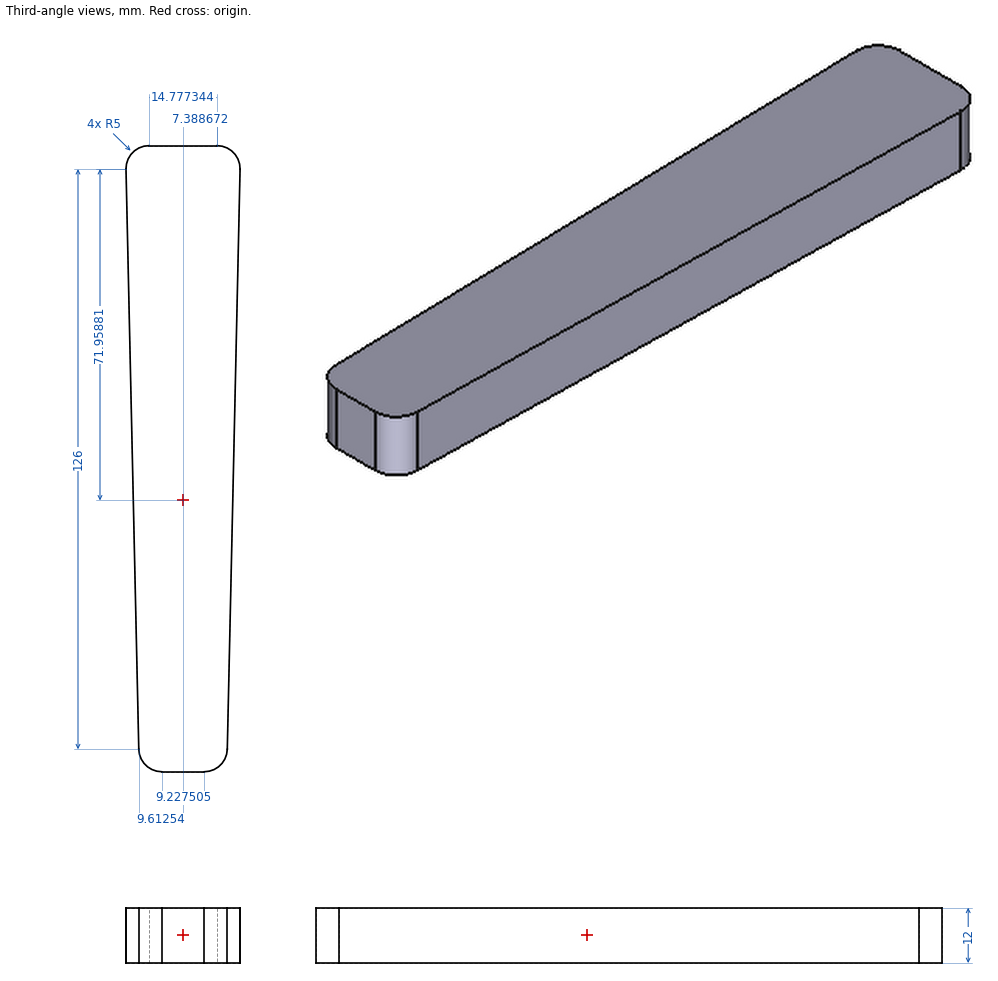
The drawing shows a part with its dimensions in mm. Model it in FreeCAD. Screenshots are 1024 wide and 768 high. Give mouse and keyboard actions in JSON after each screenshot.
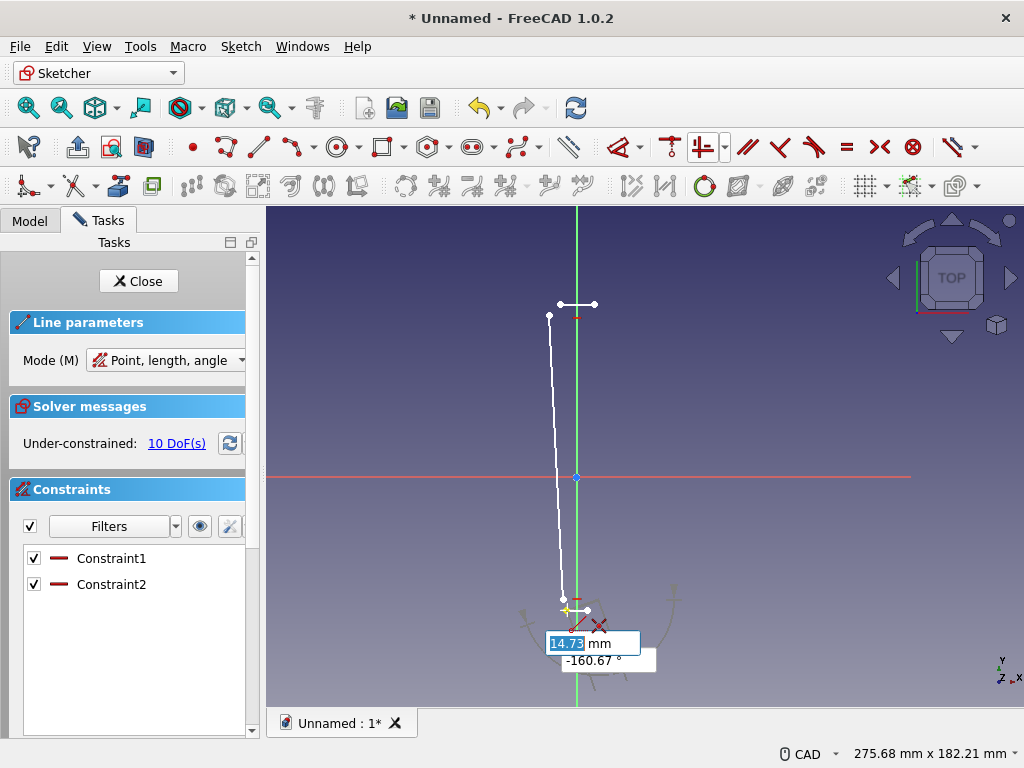
{"action": "left_click", "coordinate": [613, 315]}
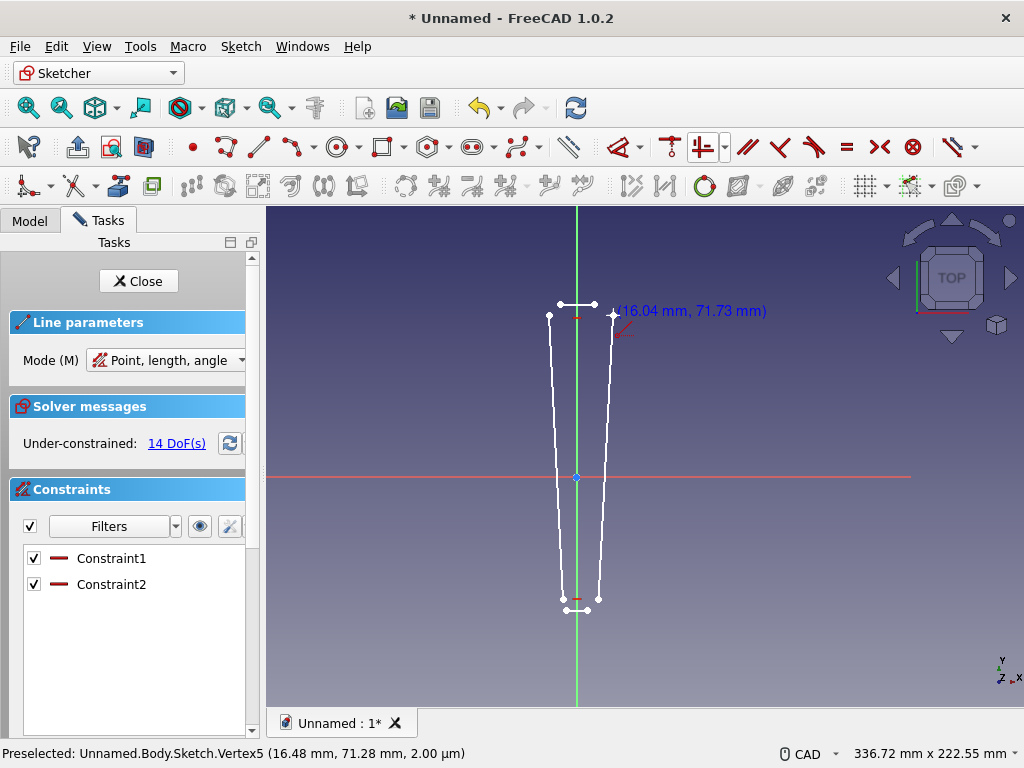
{"action": "key", "text": "g 3 a"}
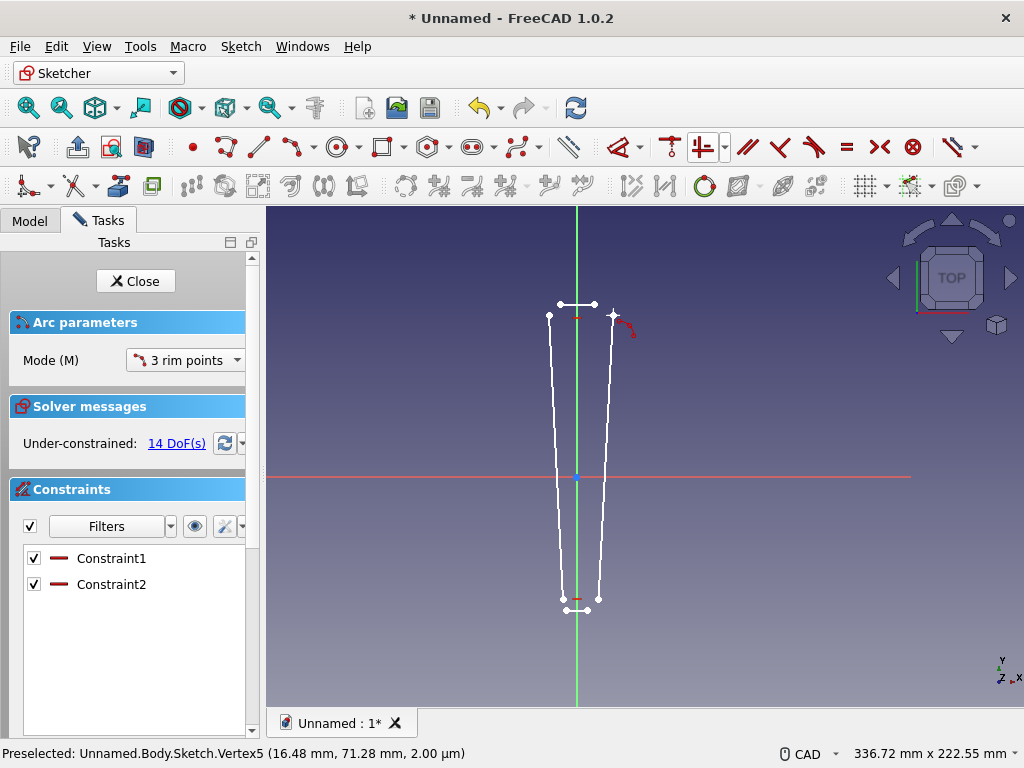
{"action": "left_click", "coordinate": [560, 305]}
{"action": "left_click", "coordinate": [549, 316]}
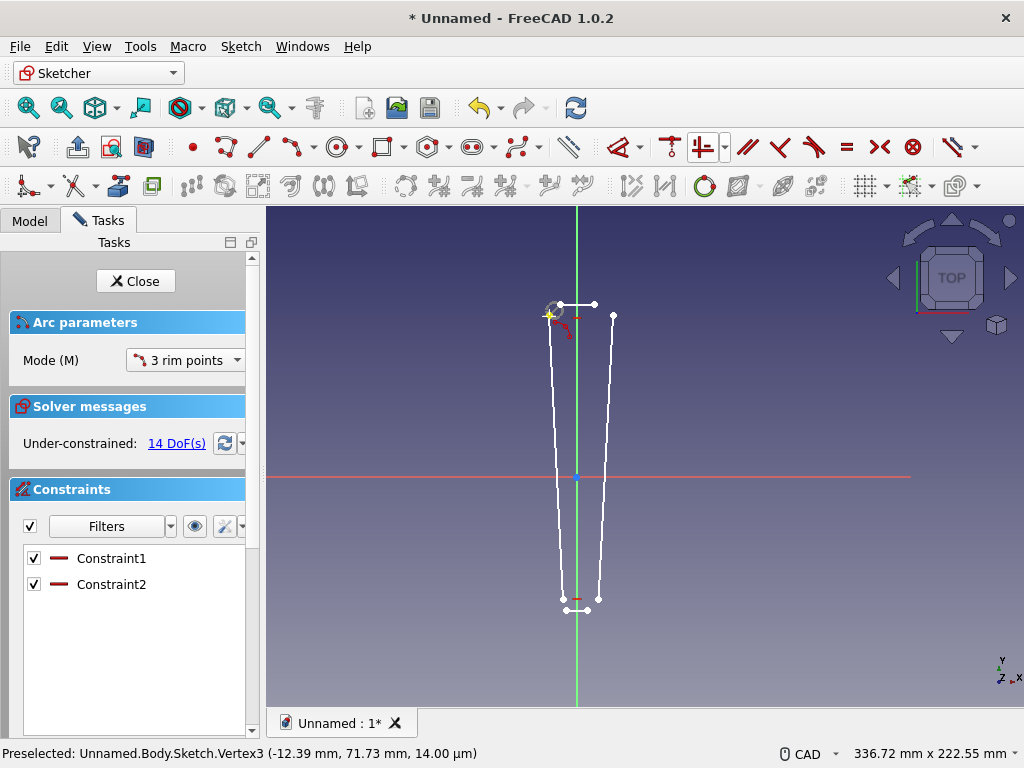
{"action": "scroll", "coordinate": [552, 307], "scroll_direction": "up", "scroll_amount": 8}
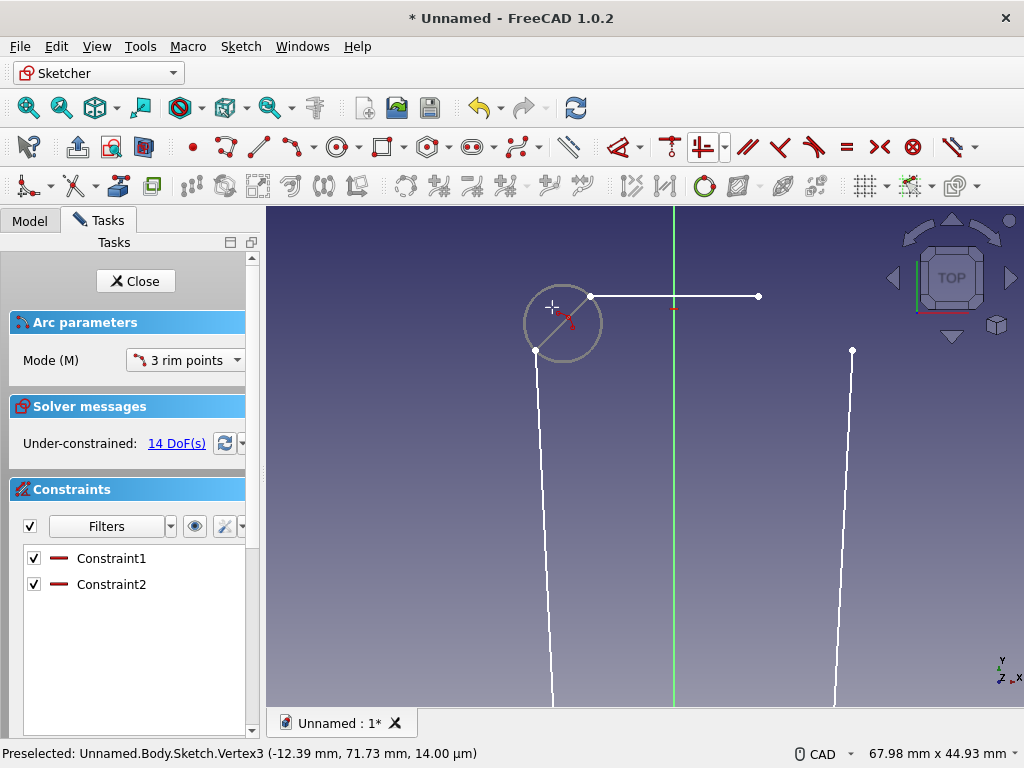
{"action": "left_click", "coordinate": [552, 308]}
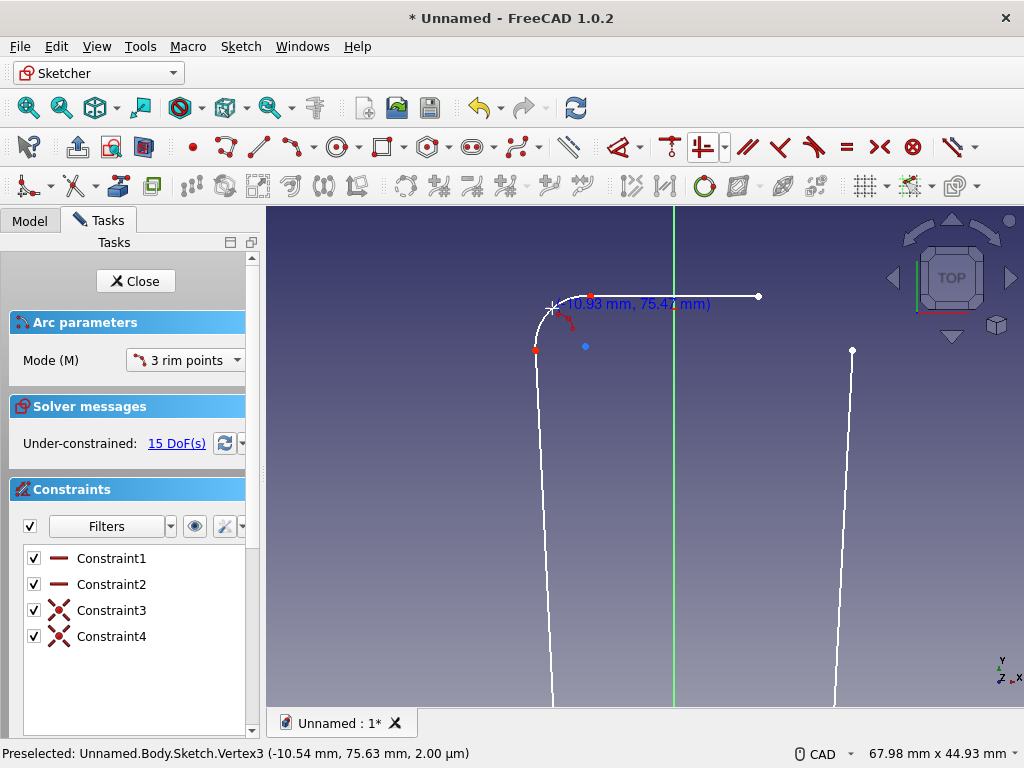
{"action": "scroll", "coordinate": [552, 307], "scroll_direction": "down", "scroll_amount": 8}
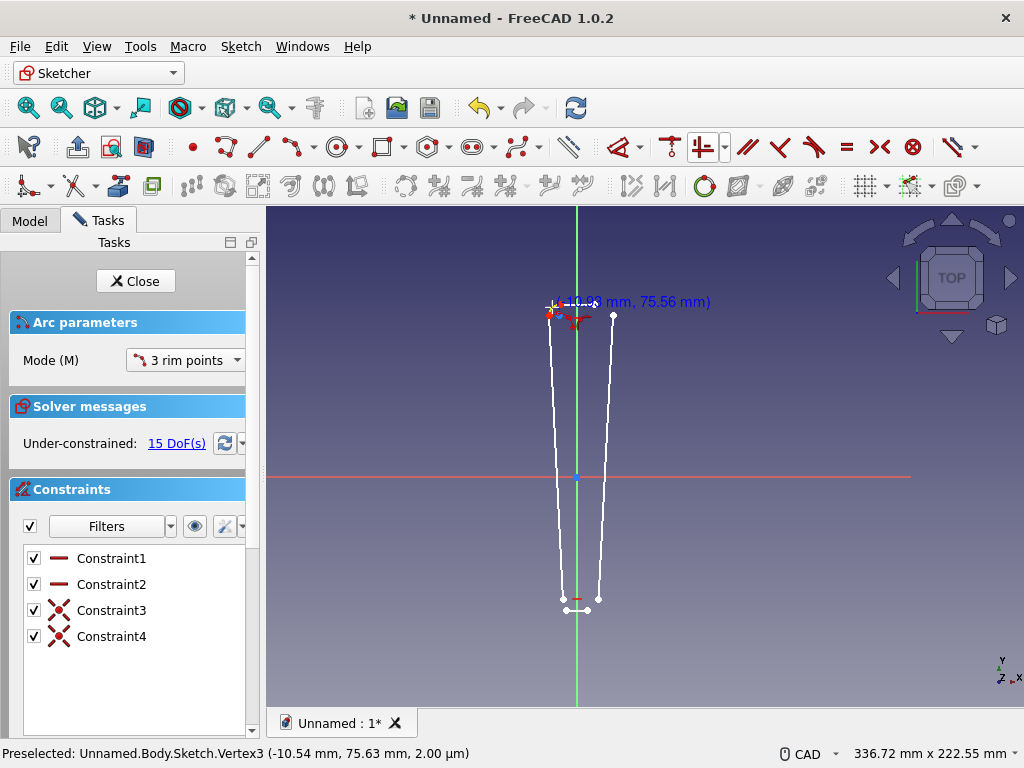
{"action": "left_click", "coordinate": [563, 600]}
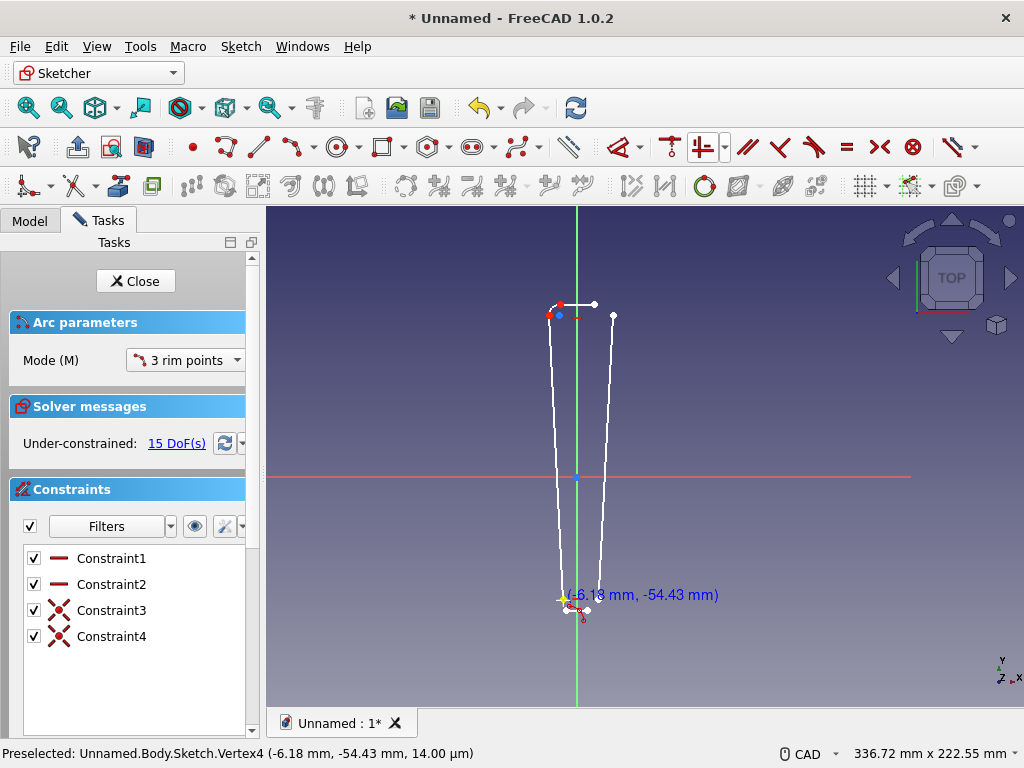
{"action": "scroll", "coordinate": [567, 610], "scroll_direction": "up", "scroll_amount": 3}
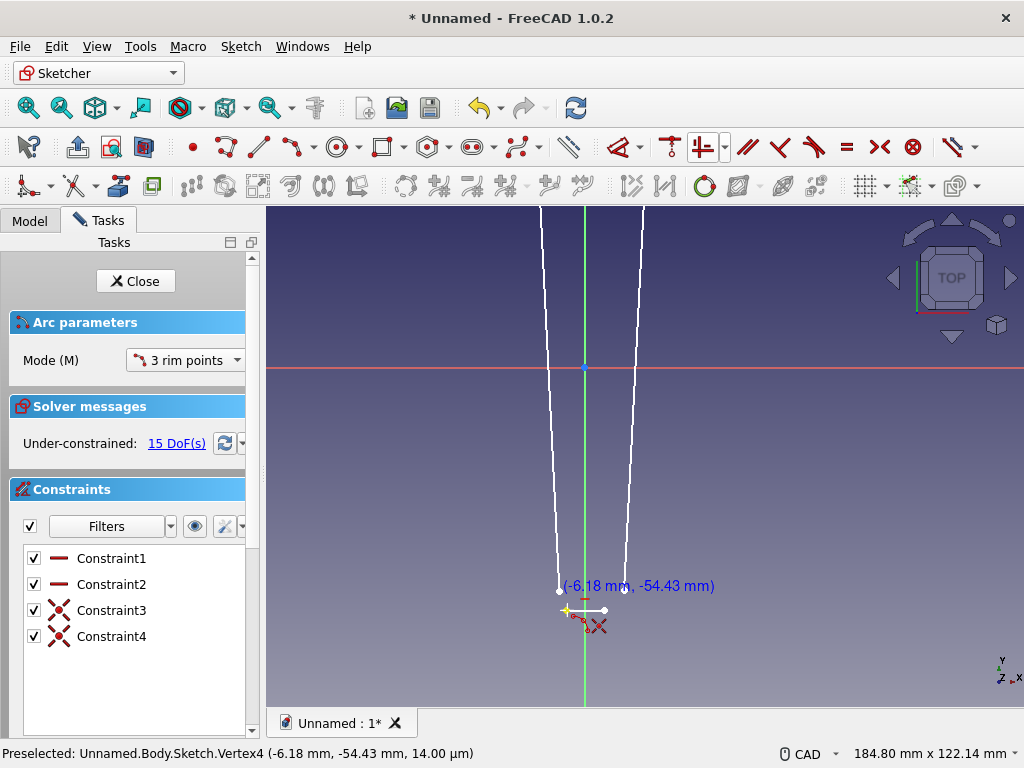
{"action": "left_click", "coordinate": [566, 611]}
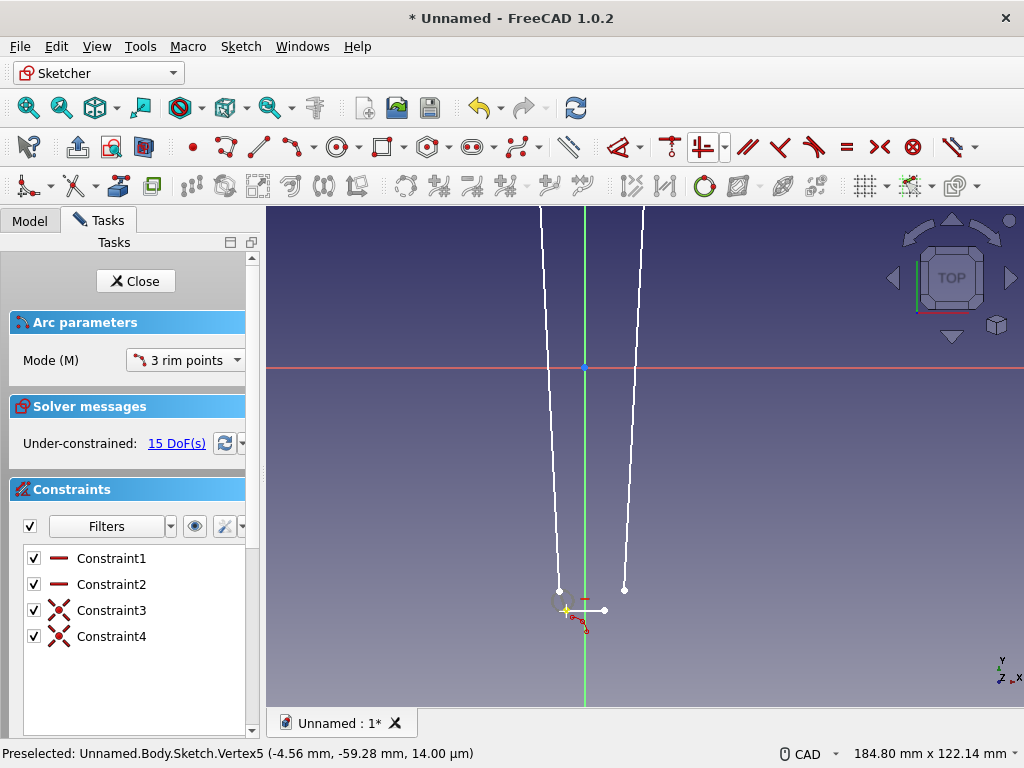
{"action": "scroll", "coordinate": [551, 604], "scroll_direction": "up", "scroll_amount": 5}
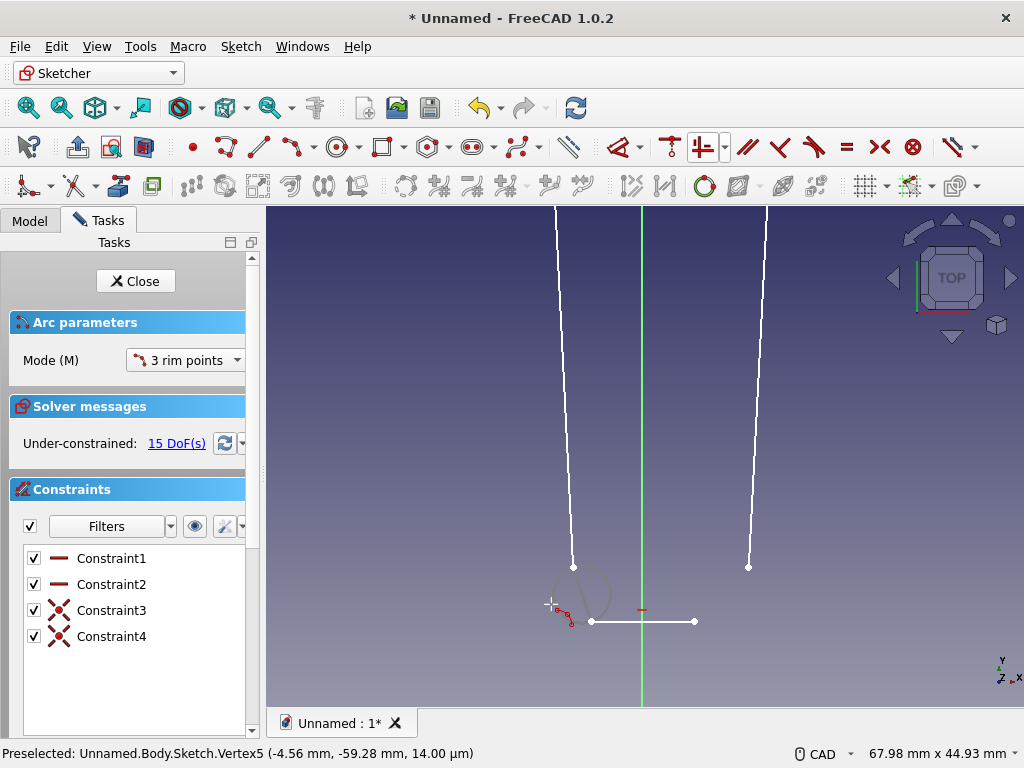
{"action": "left_click", "coordinate": [552, 602]}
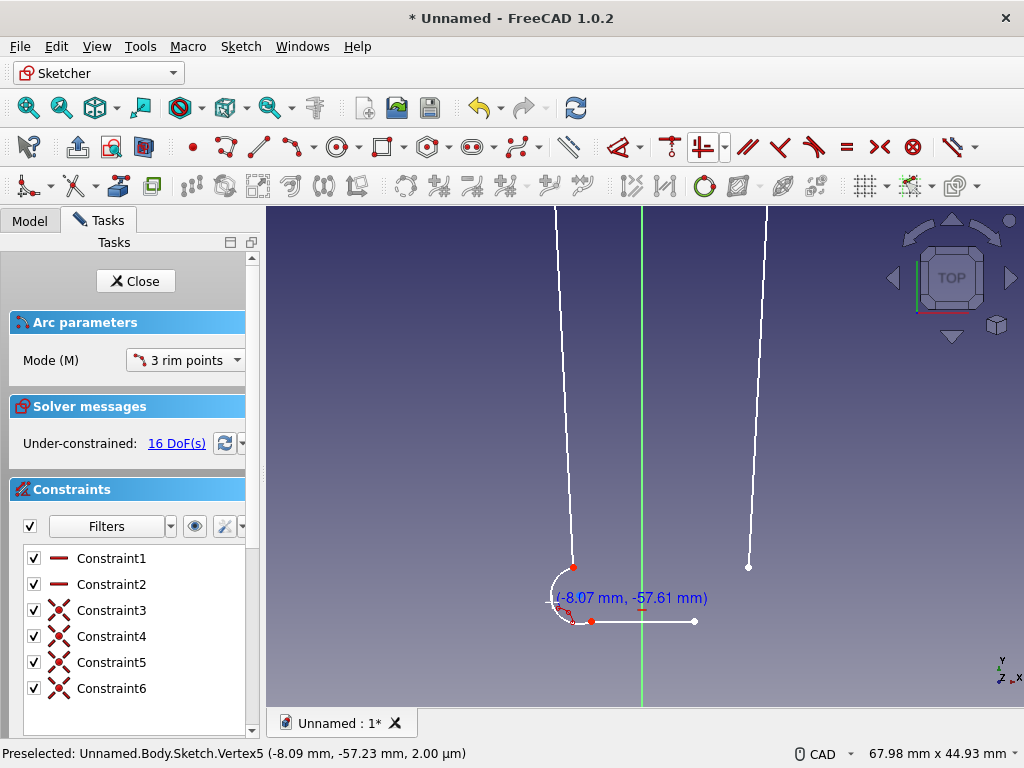
{"action": "scroll", "coordinate": [560, 608], "scroll_direction": "down", "scroll_amount": 8}